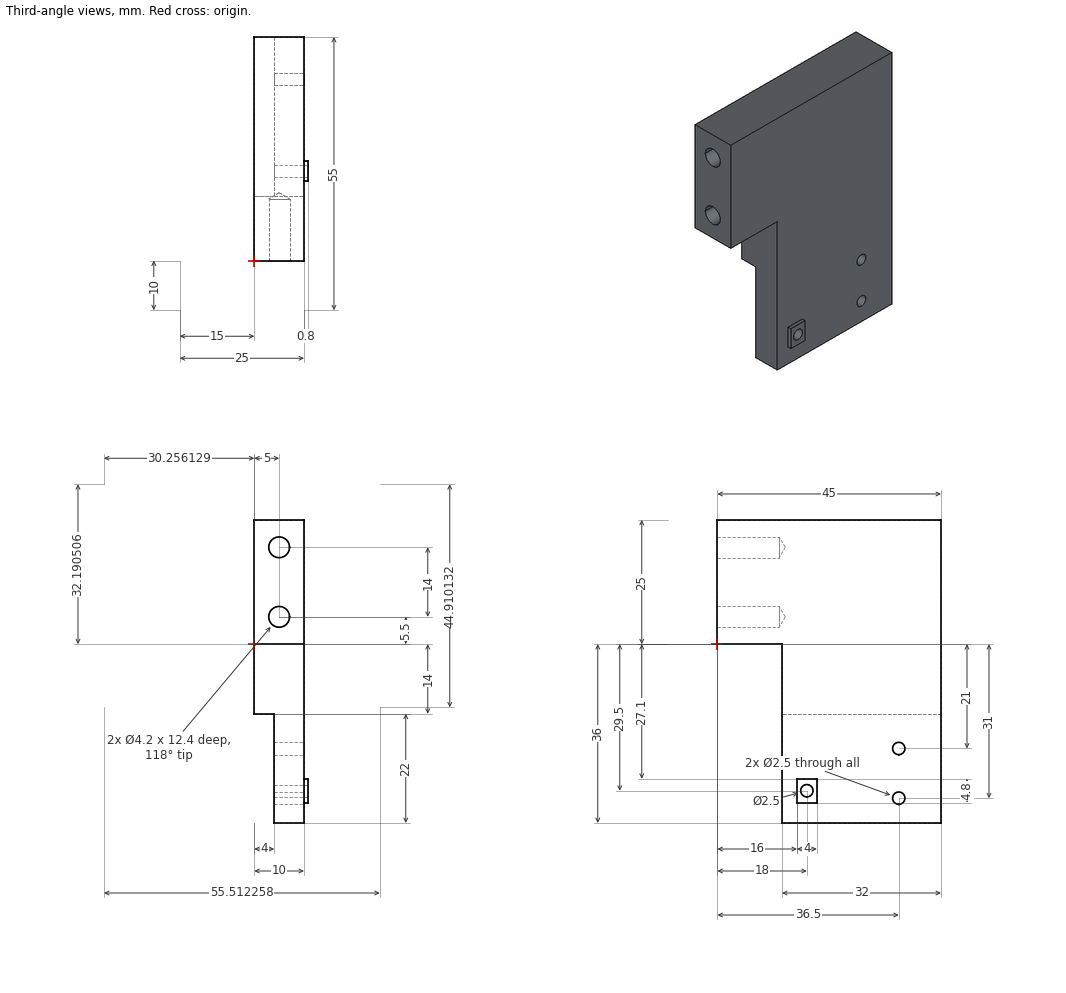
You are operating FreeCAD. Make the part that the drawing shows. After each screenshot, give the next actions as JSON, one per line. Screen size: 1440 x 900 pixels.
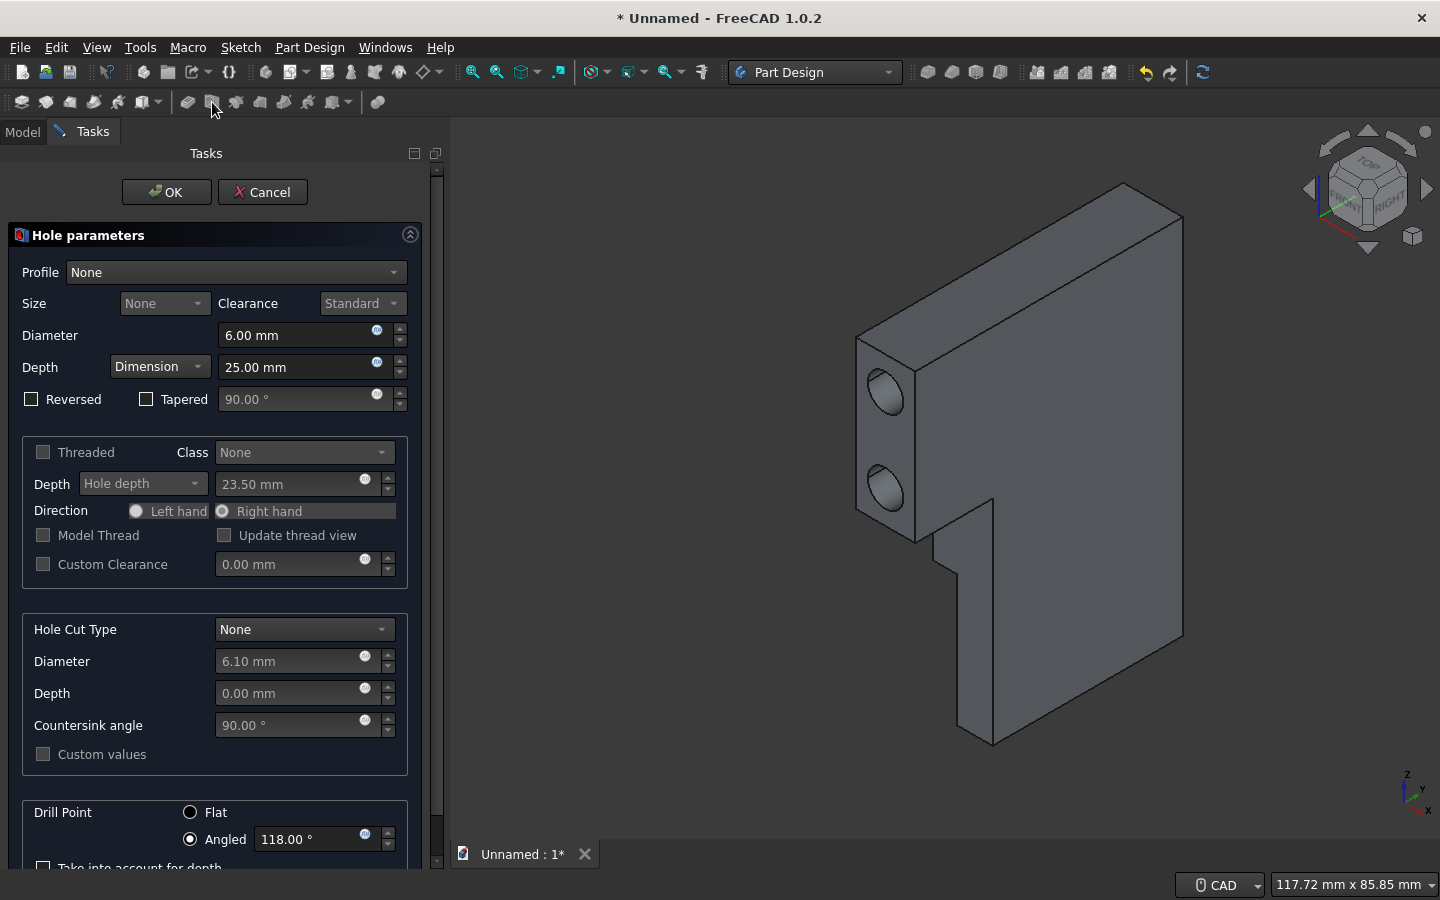
{"action": "triple_click", "coordinate": [305, 335]}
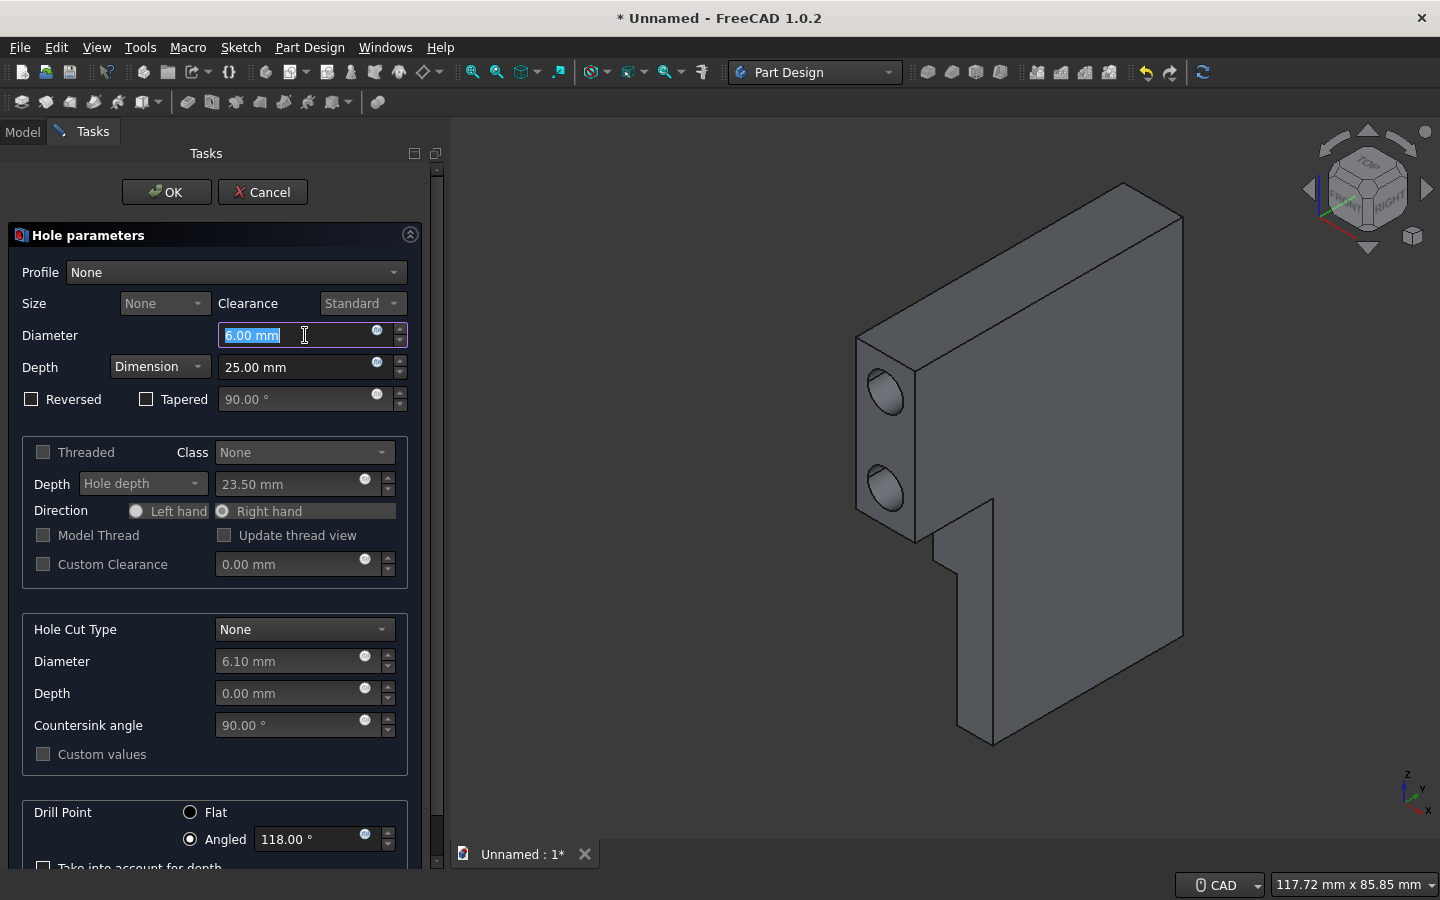
{"action": "type", "text": "4.2"}
{"action": "key", "text": "Tab"}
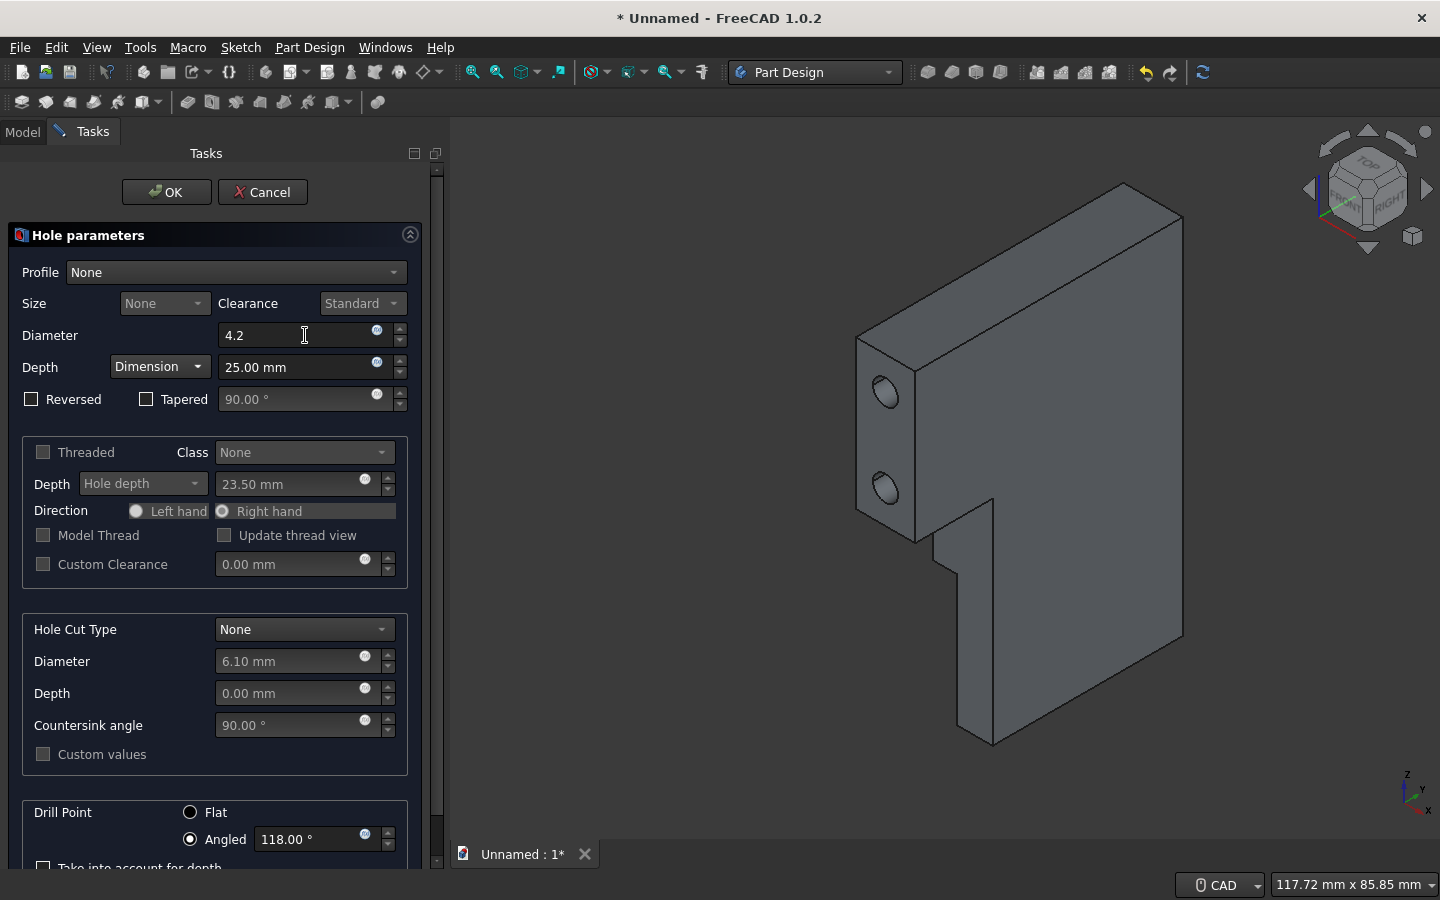
{"action": "triple_click", "coordinate": [305, 367]}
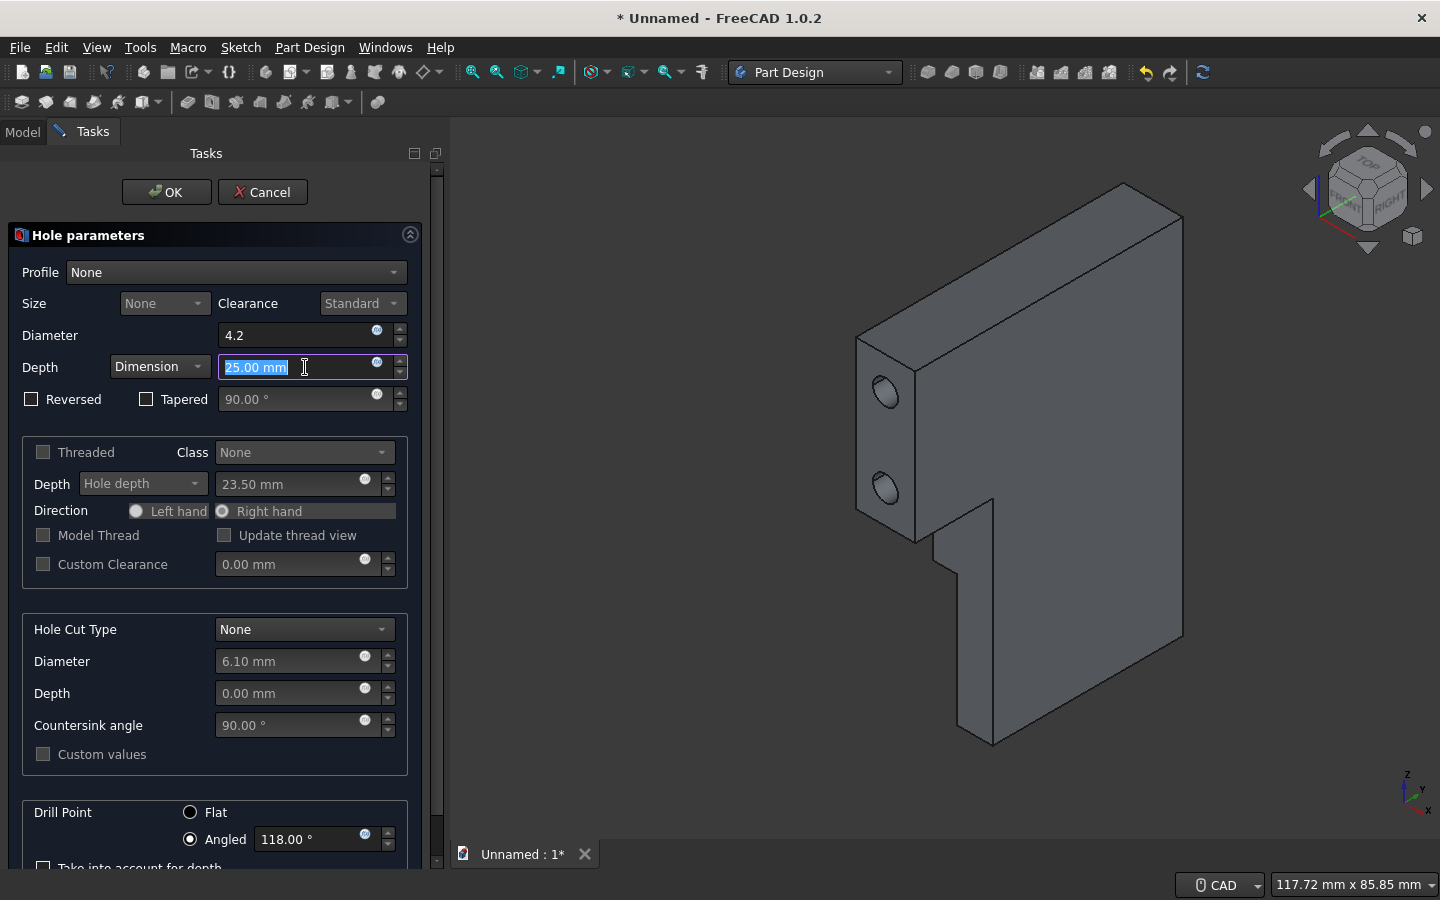
{"action": "type", "text": "12.4"}
{"action": "key", "text": "Tab"}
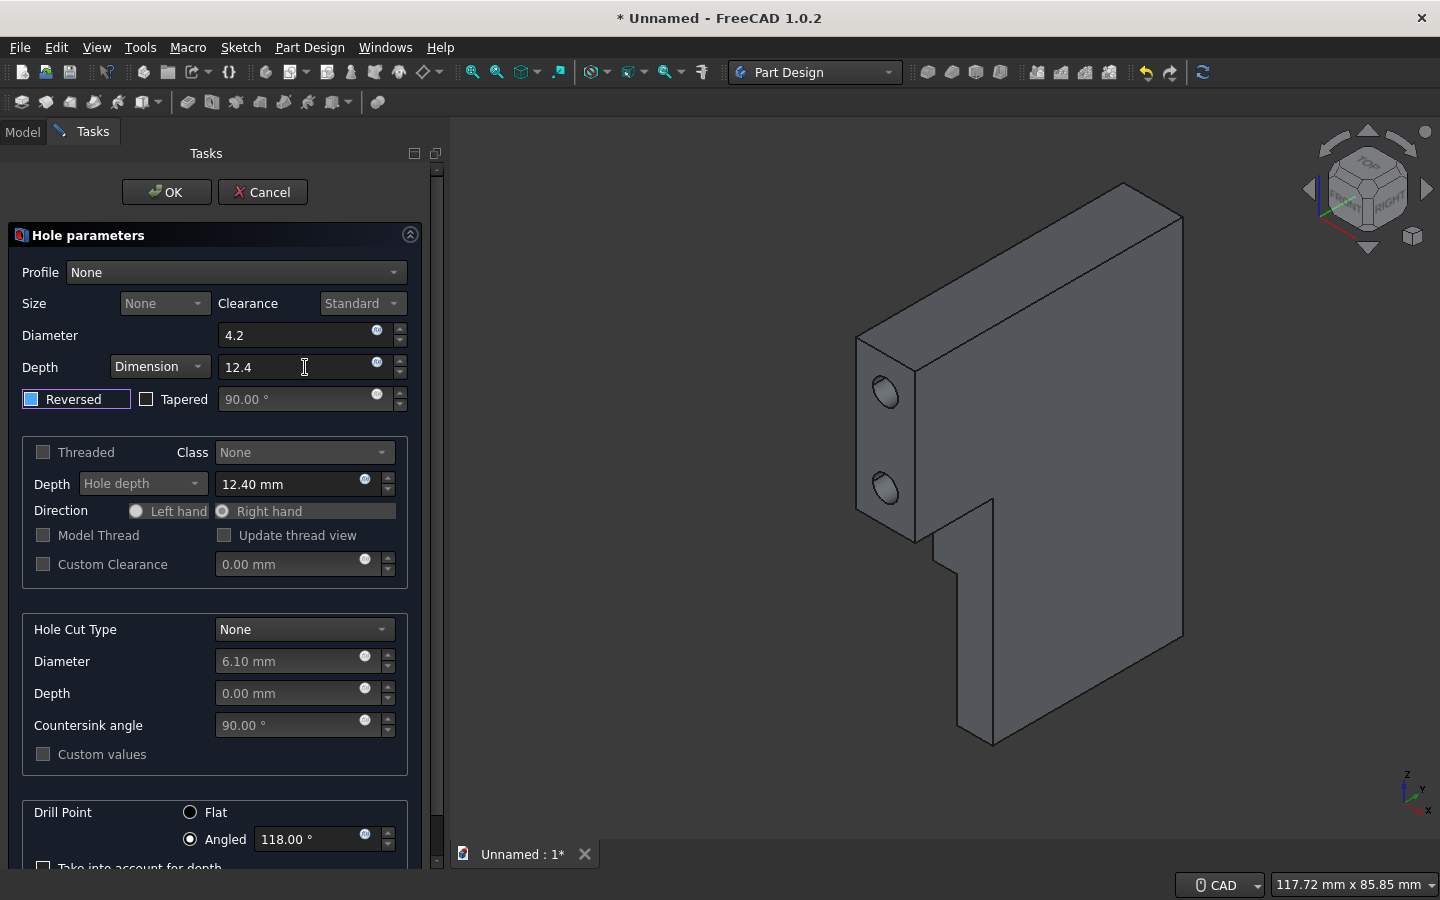
{"action": "left_click", "coordinate": [167, 192]}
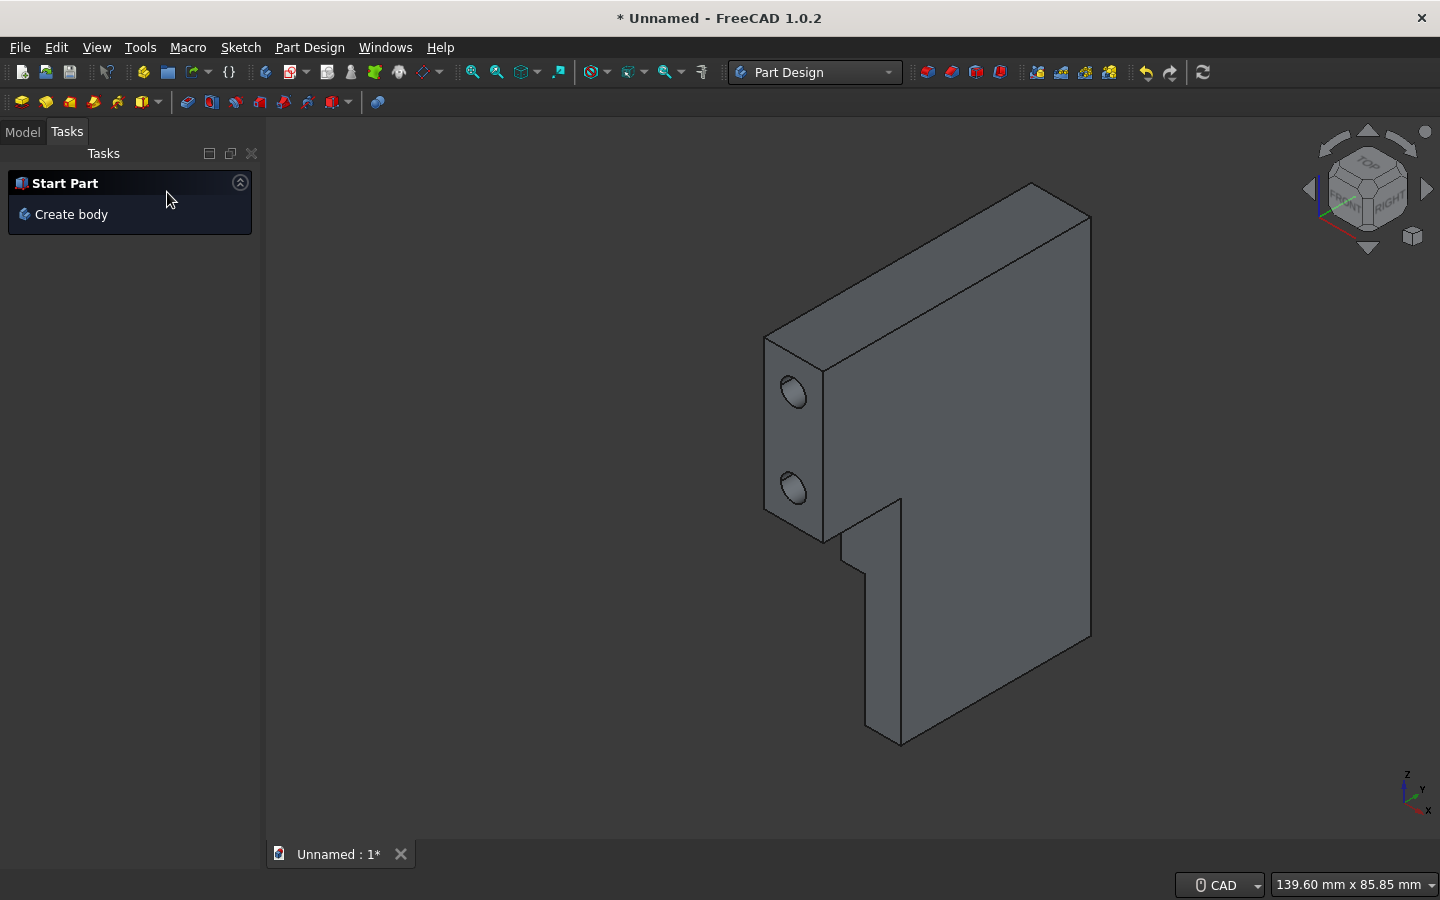
{"action": "key", "text": "6"}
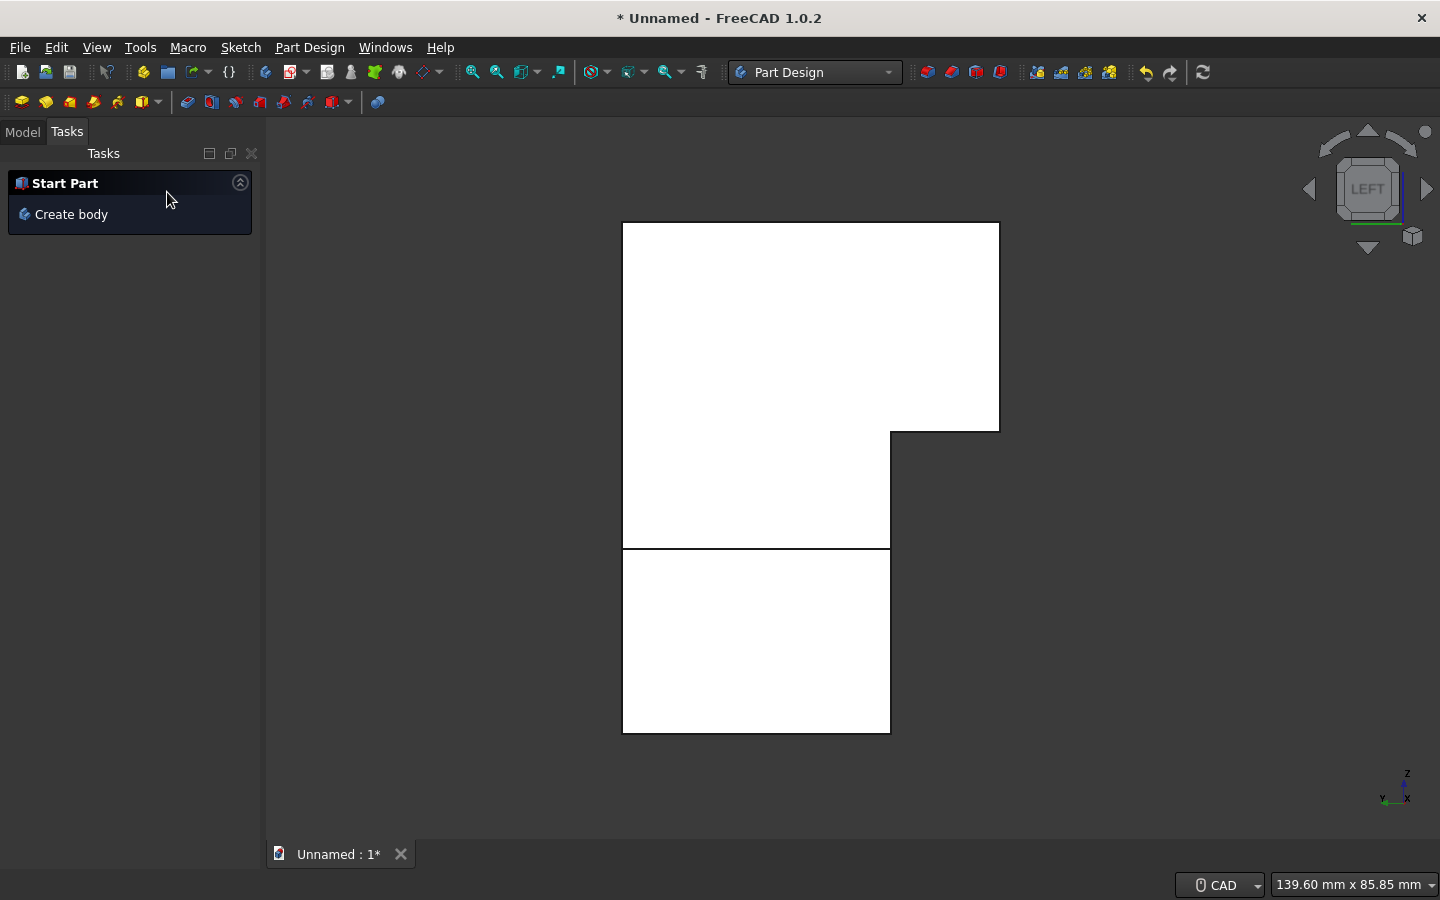
{"action": "left_click", "coordinate": [718, 641]}